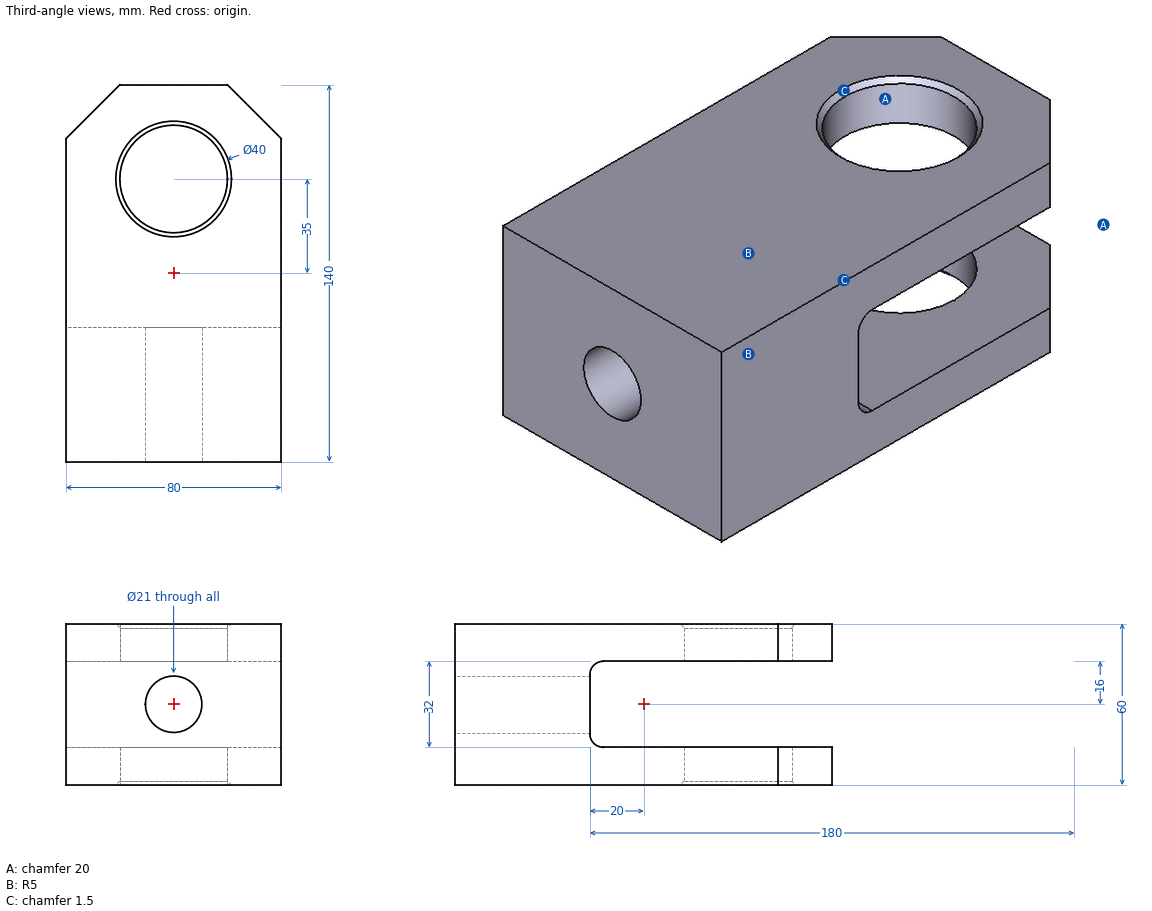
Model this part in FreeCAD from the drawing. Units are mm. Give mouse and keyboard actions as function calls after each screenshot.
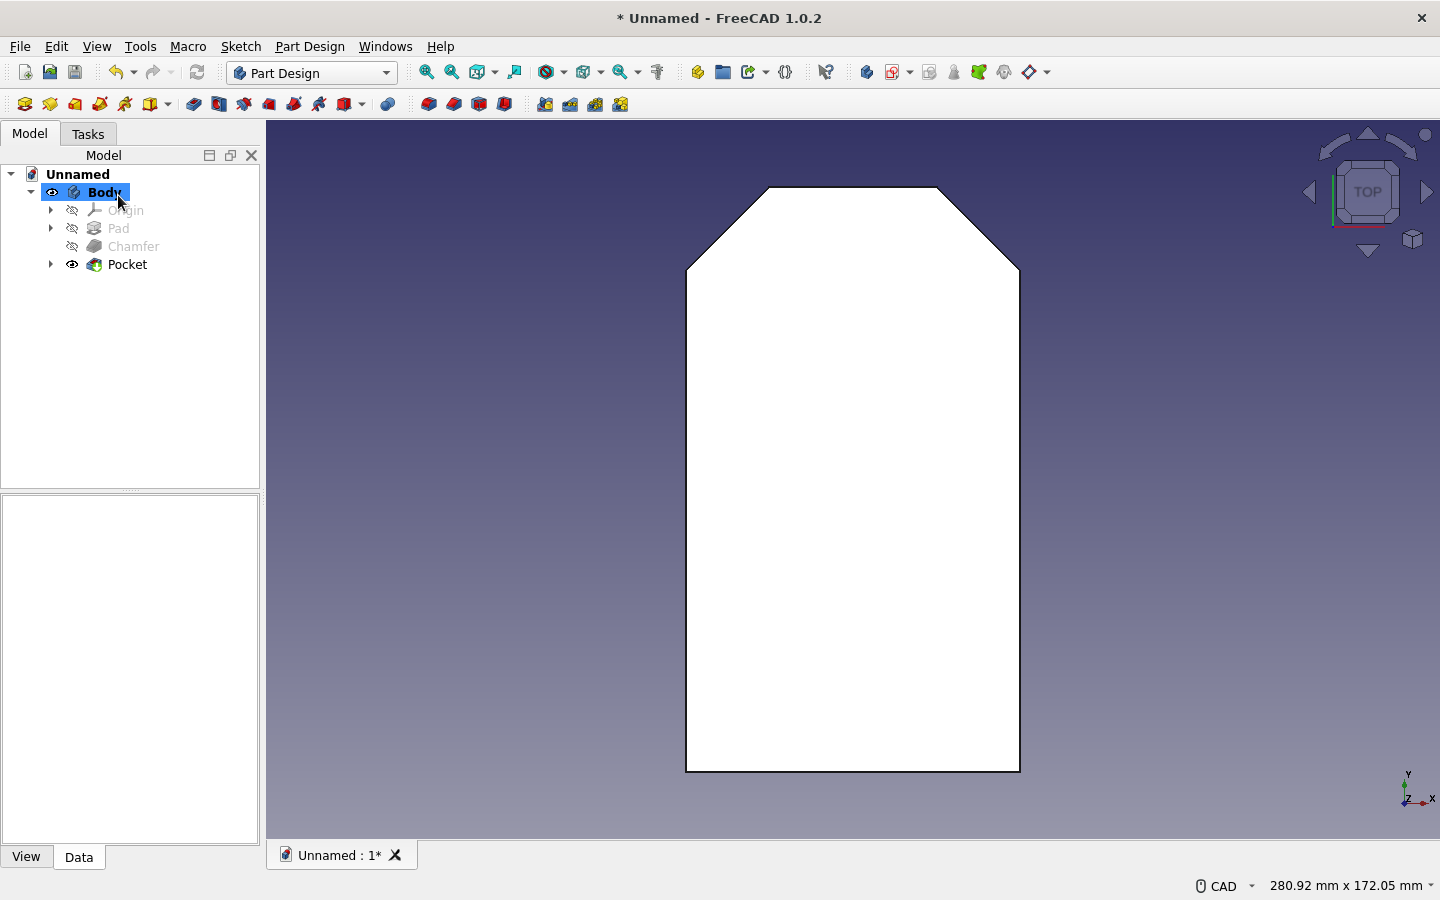
key(1)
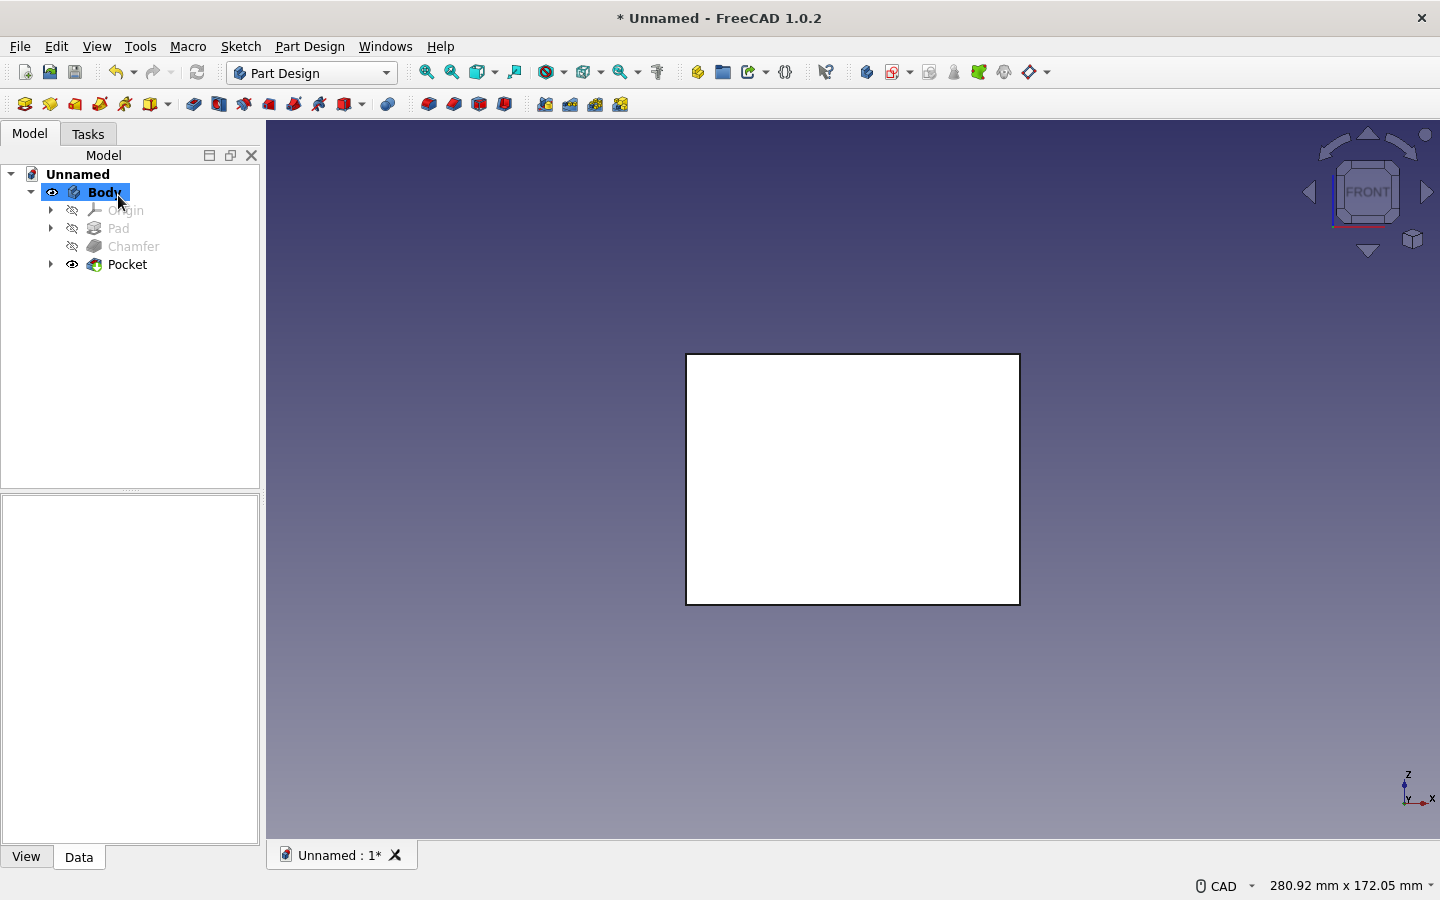
click(427, 72)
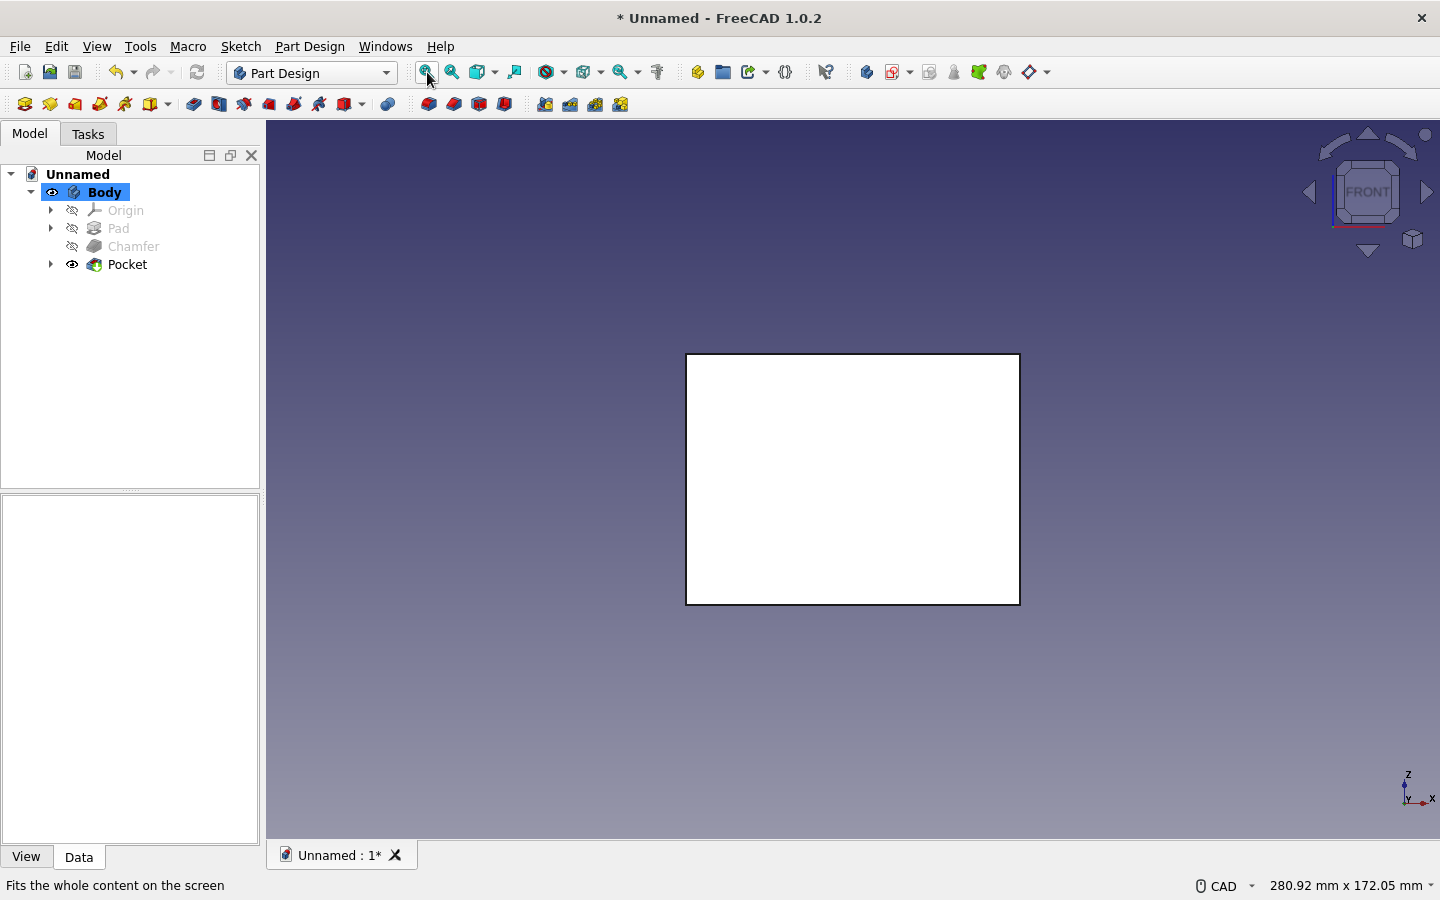
key(3)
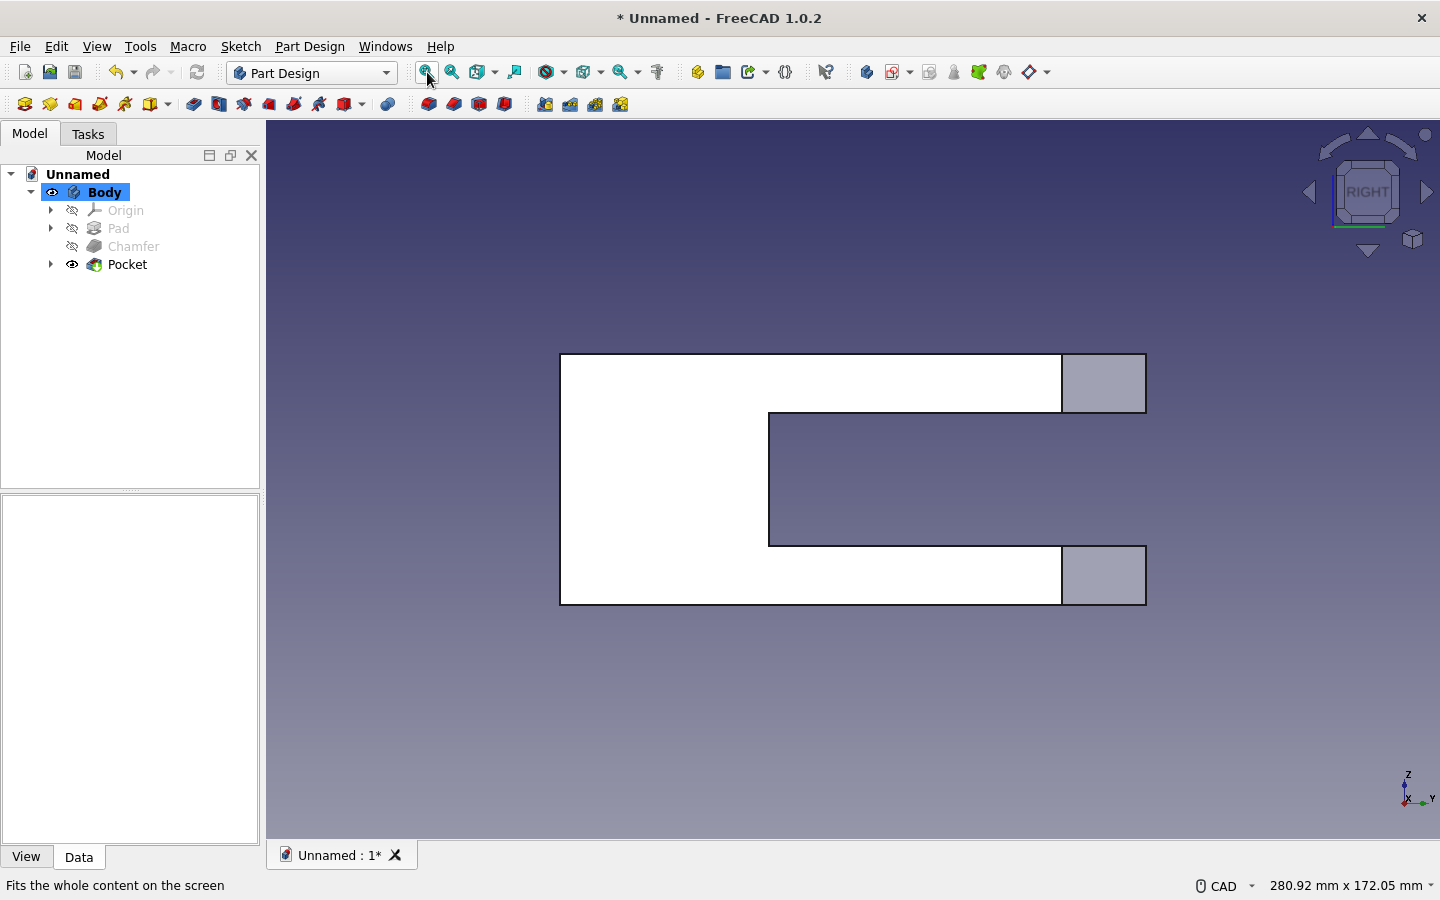
key(5)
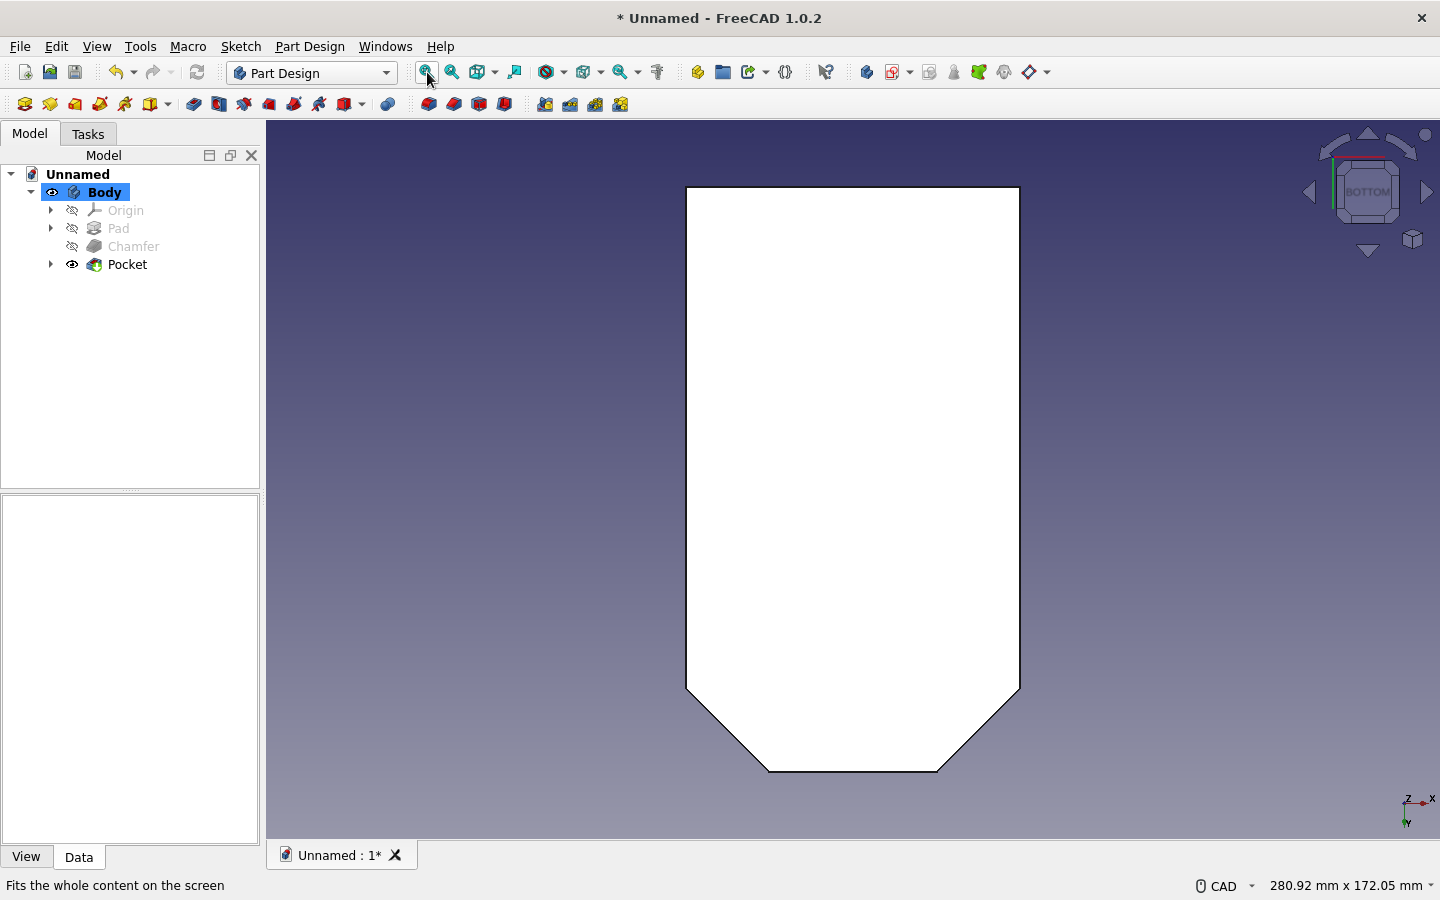
key(4)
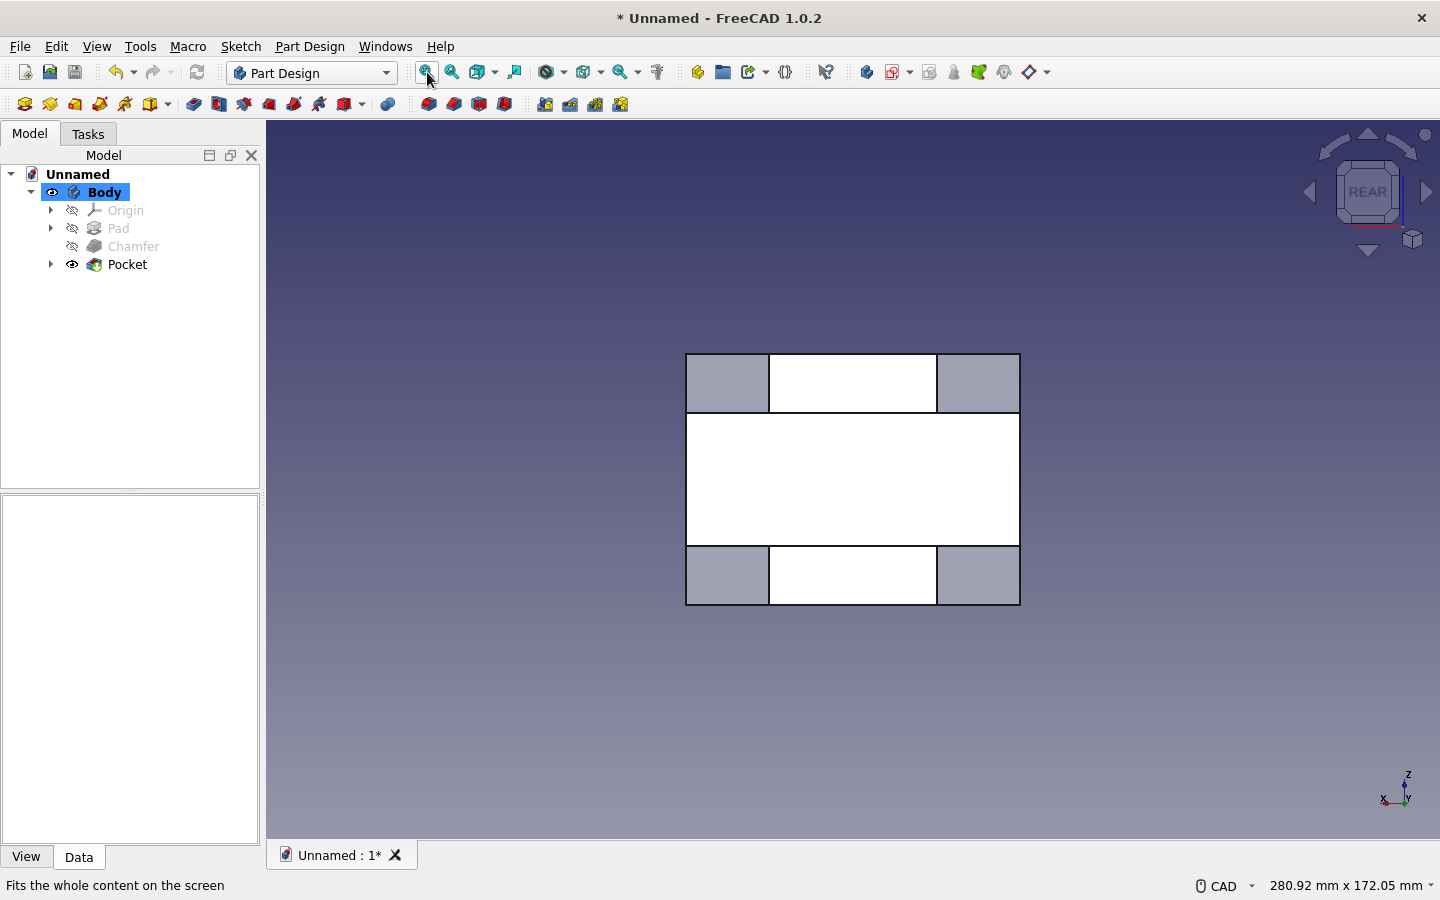
key(v)
key(f)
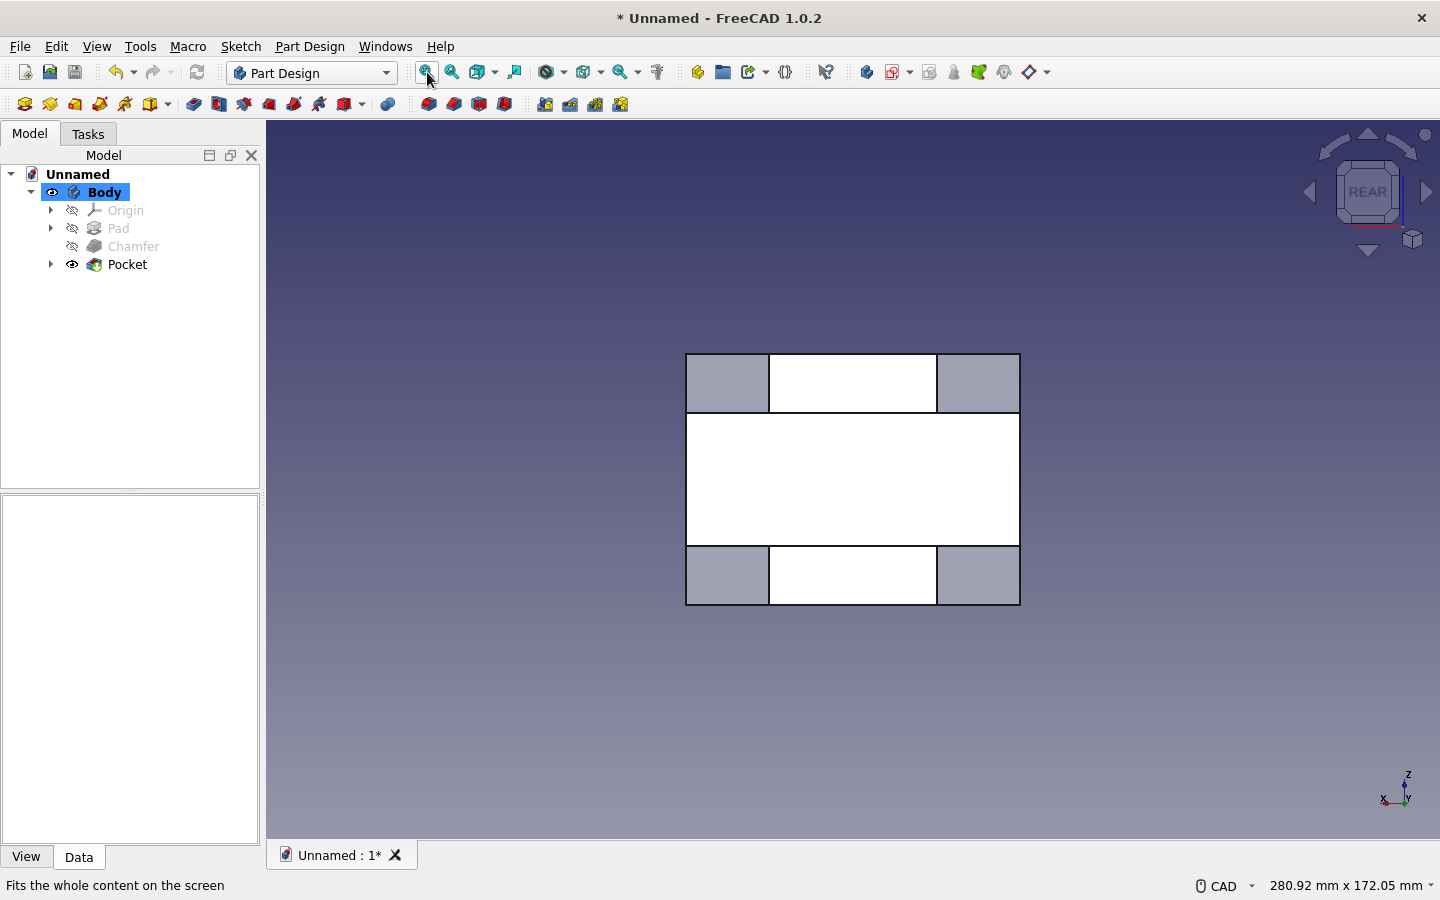
key(6)